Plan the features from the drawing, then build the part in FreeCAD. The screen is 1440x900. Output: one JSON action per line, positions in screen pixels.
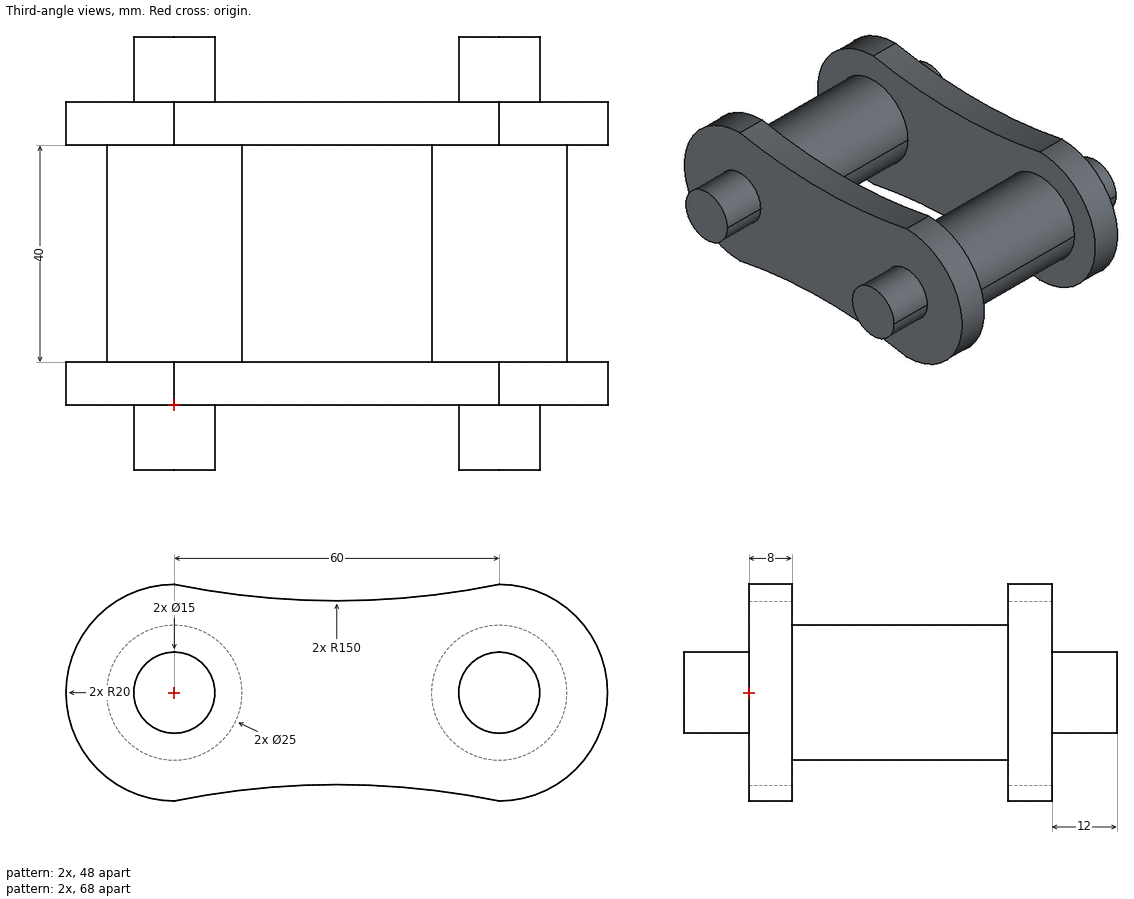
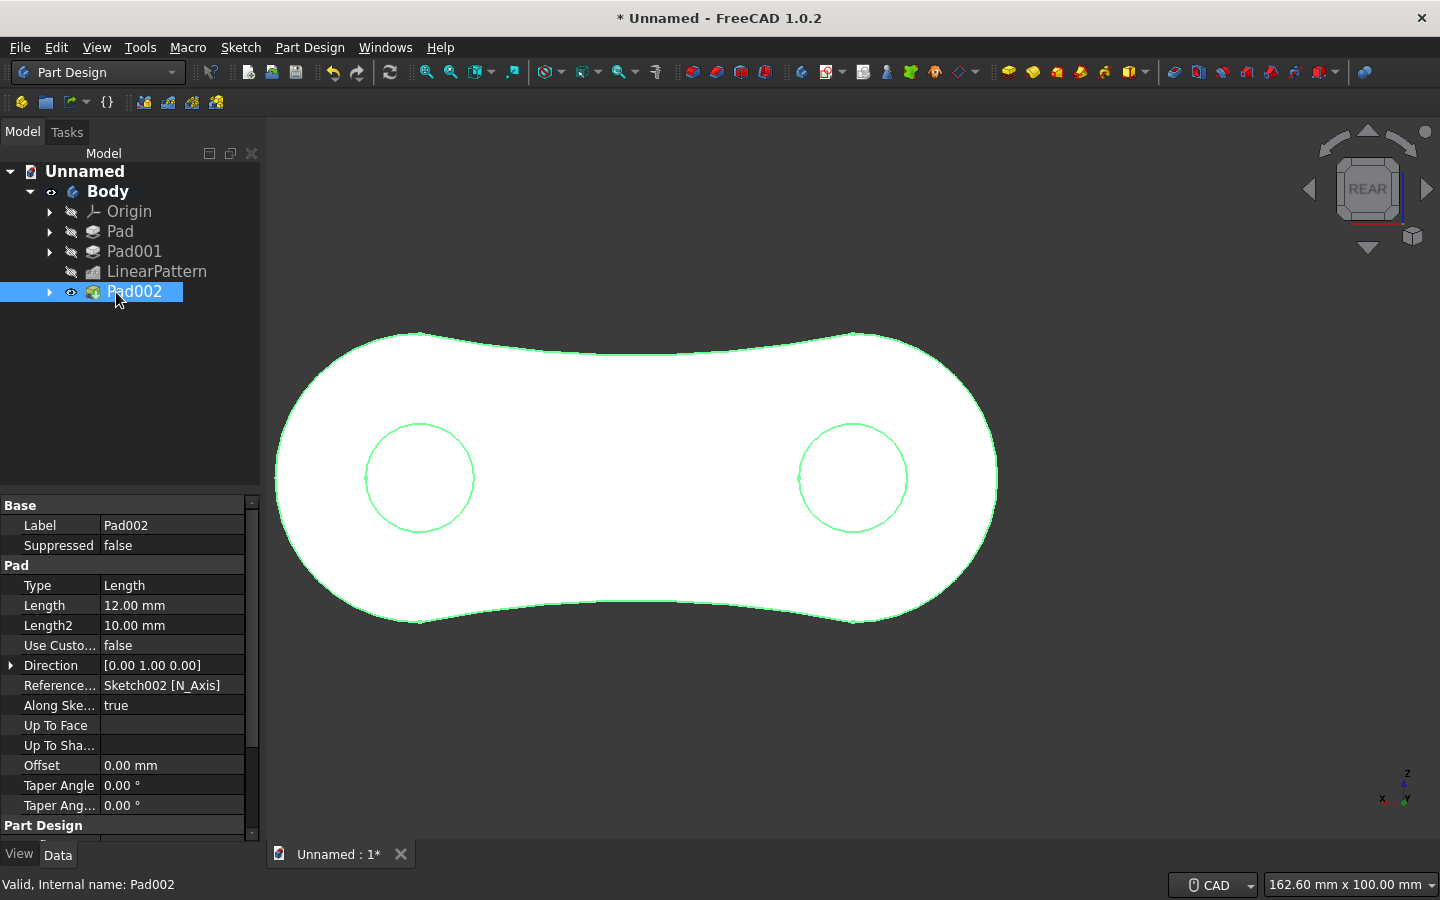
{"action": "left_click", "coordinate": [168, 102]}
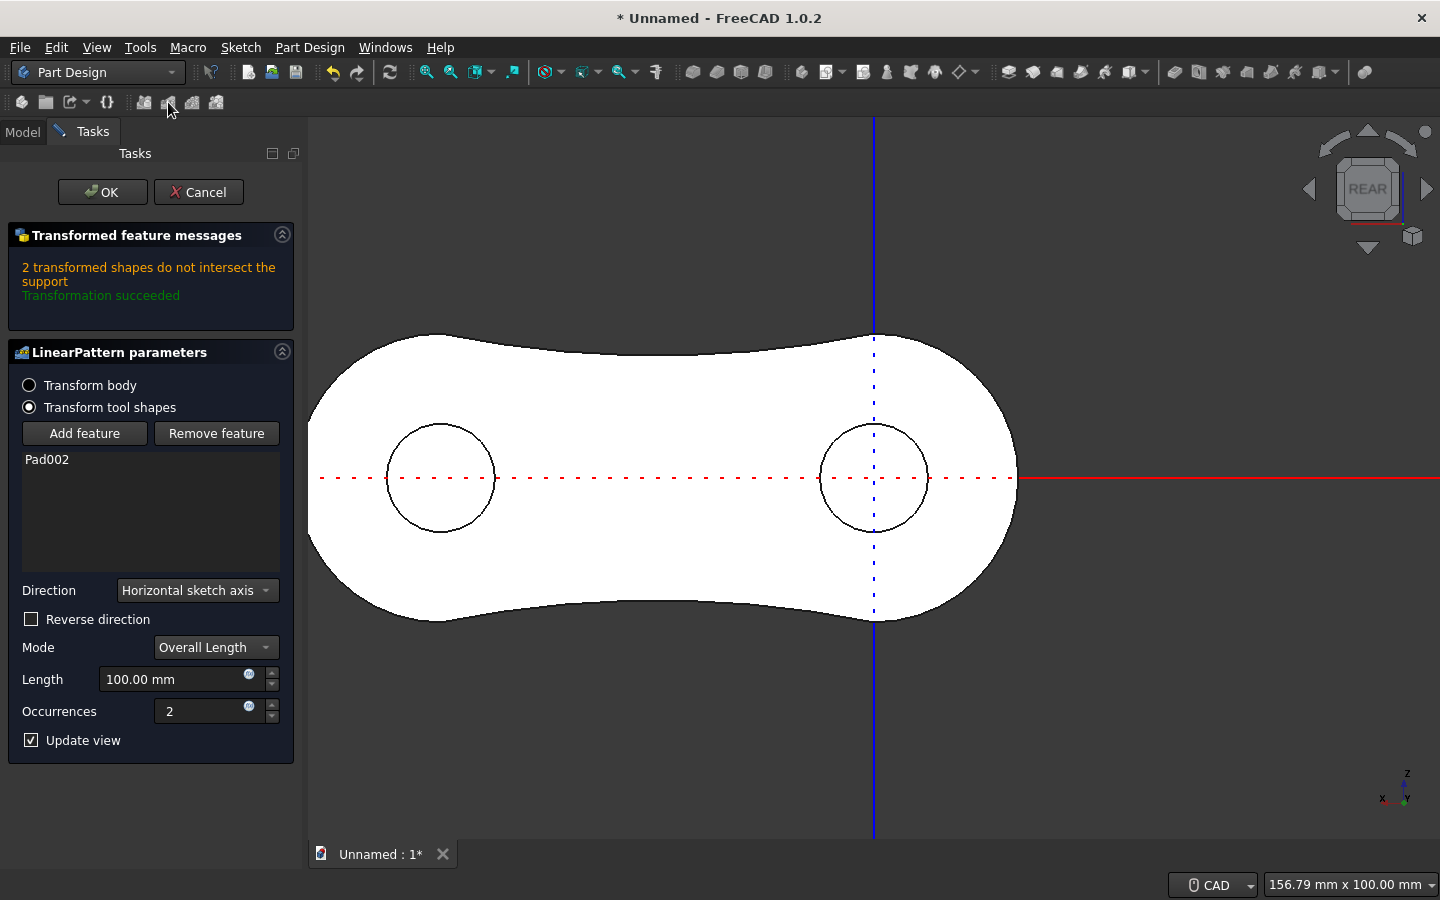
{"action": "left_click", "coordinate": [198, 590]}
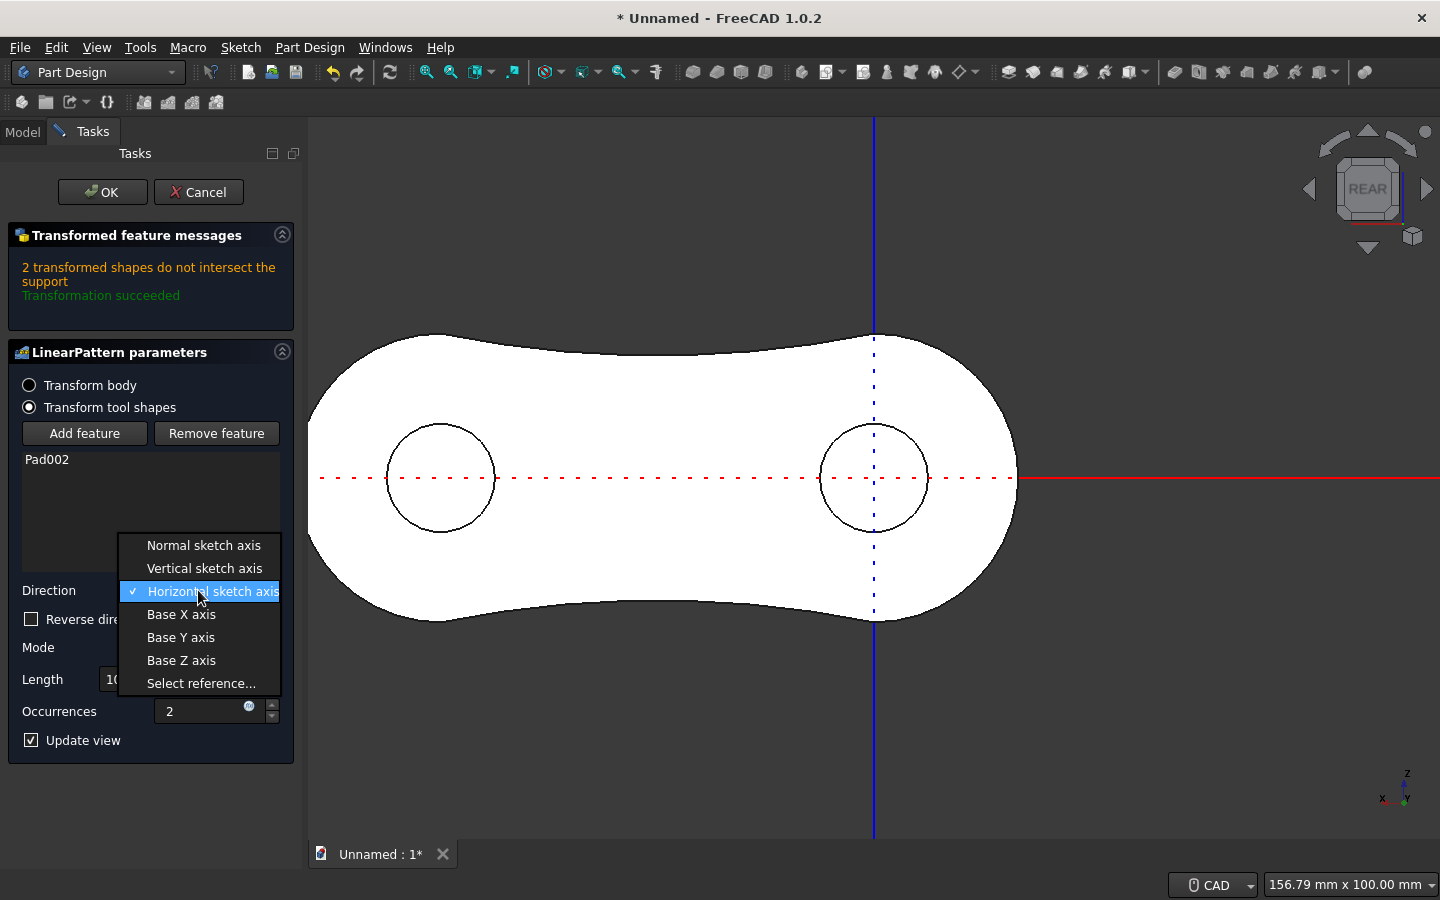
{"action": "left_click", "coordinate": [198, 638]}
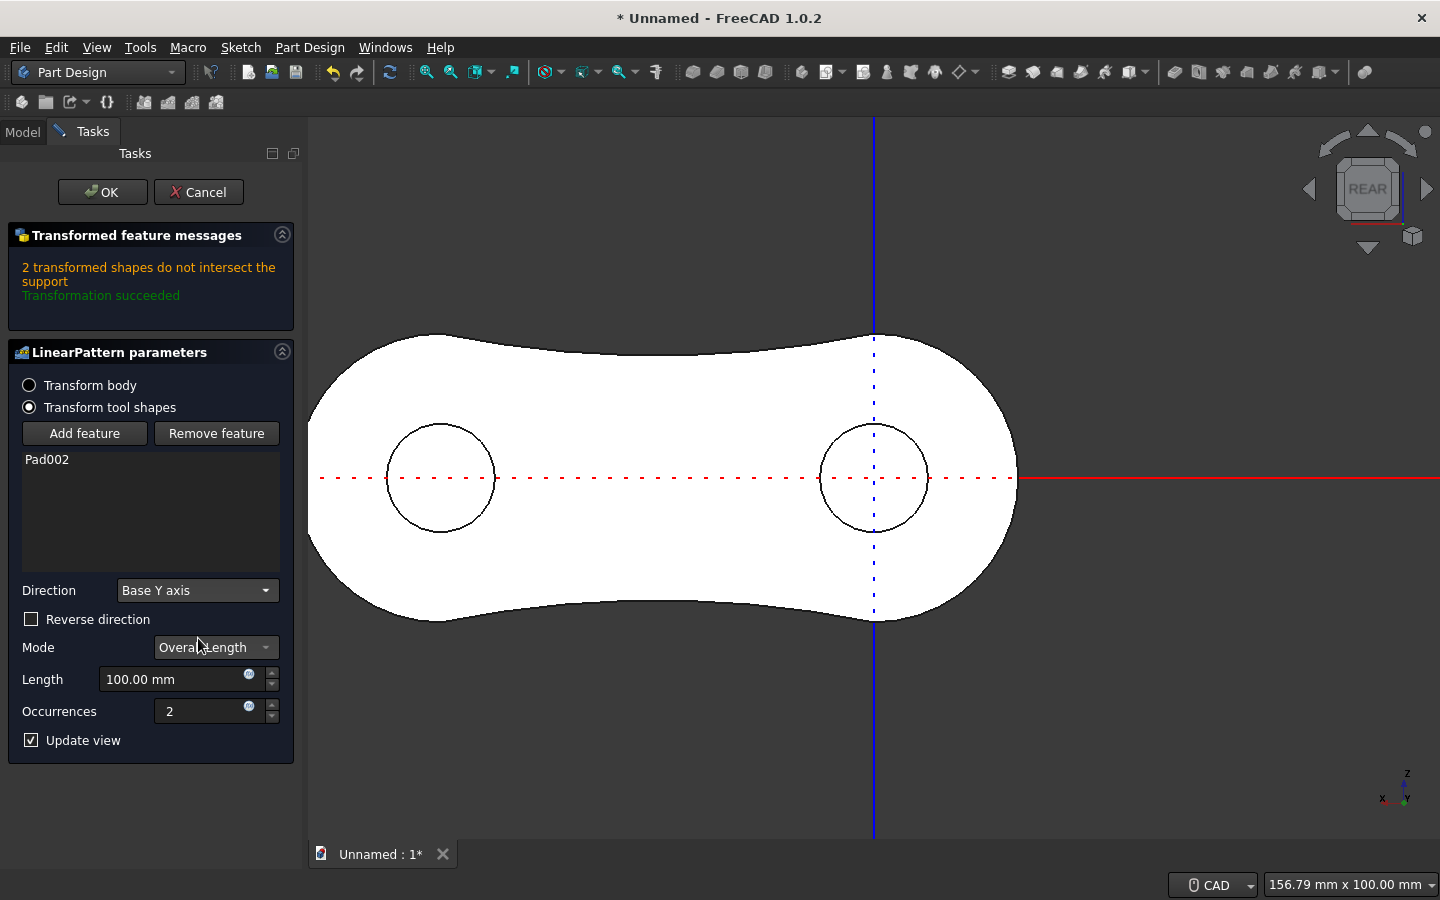
{"action": "left_click", "coordinate": [217, 648]}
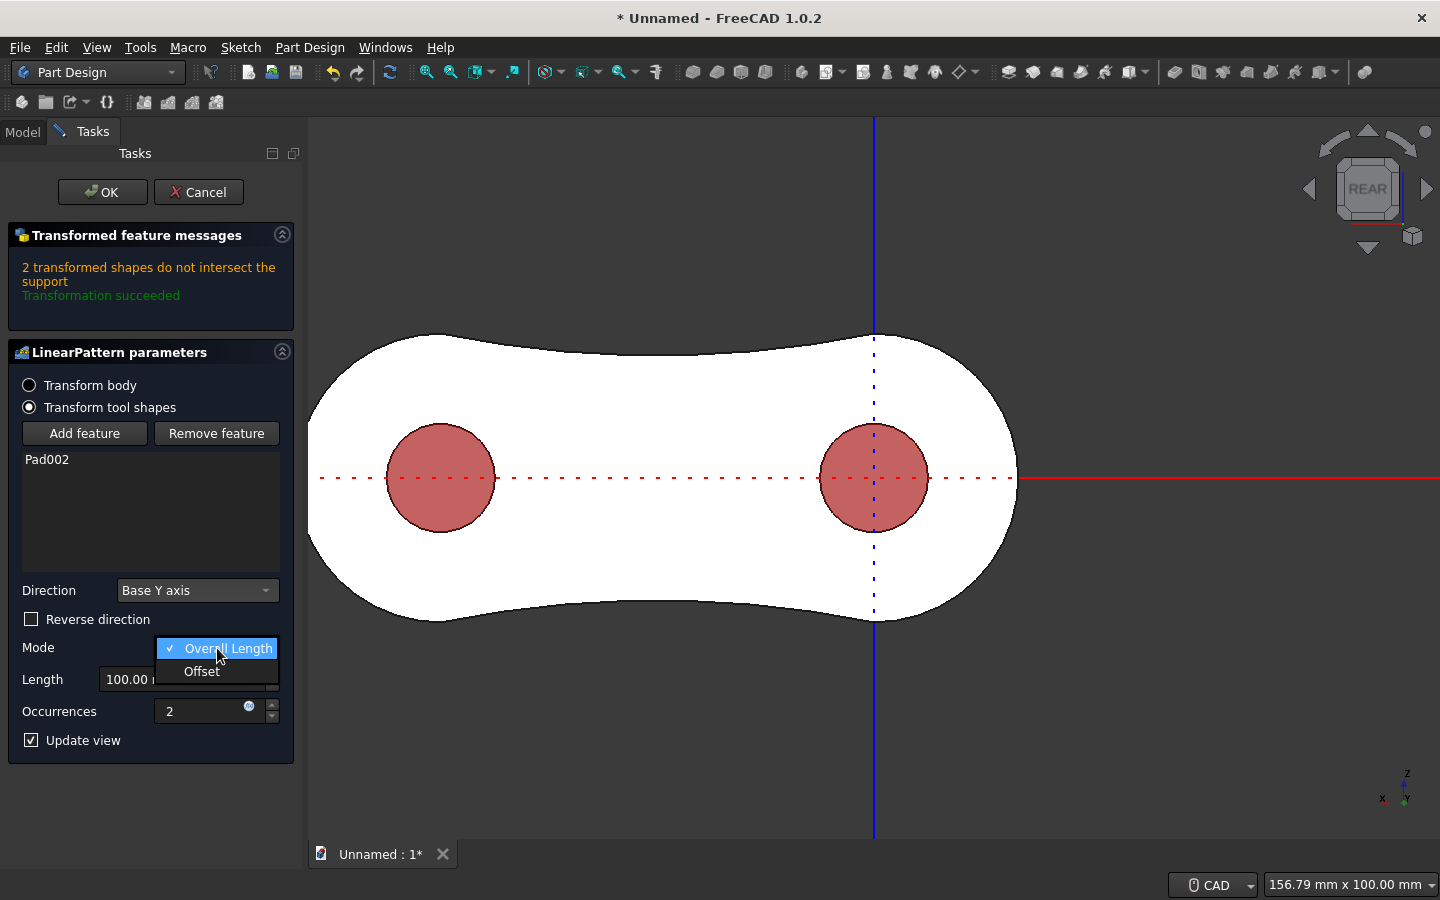
{"action": "left_click", "coordinate": [216, 672]}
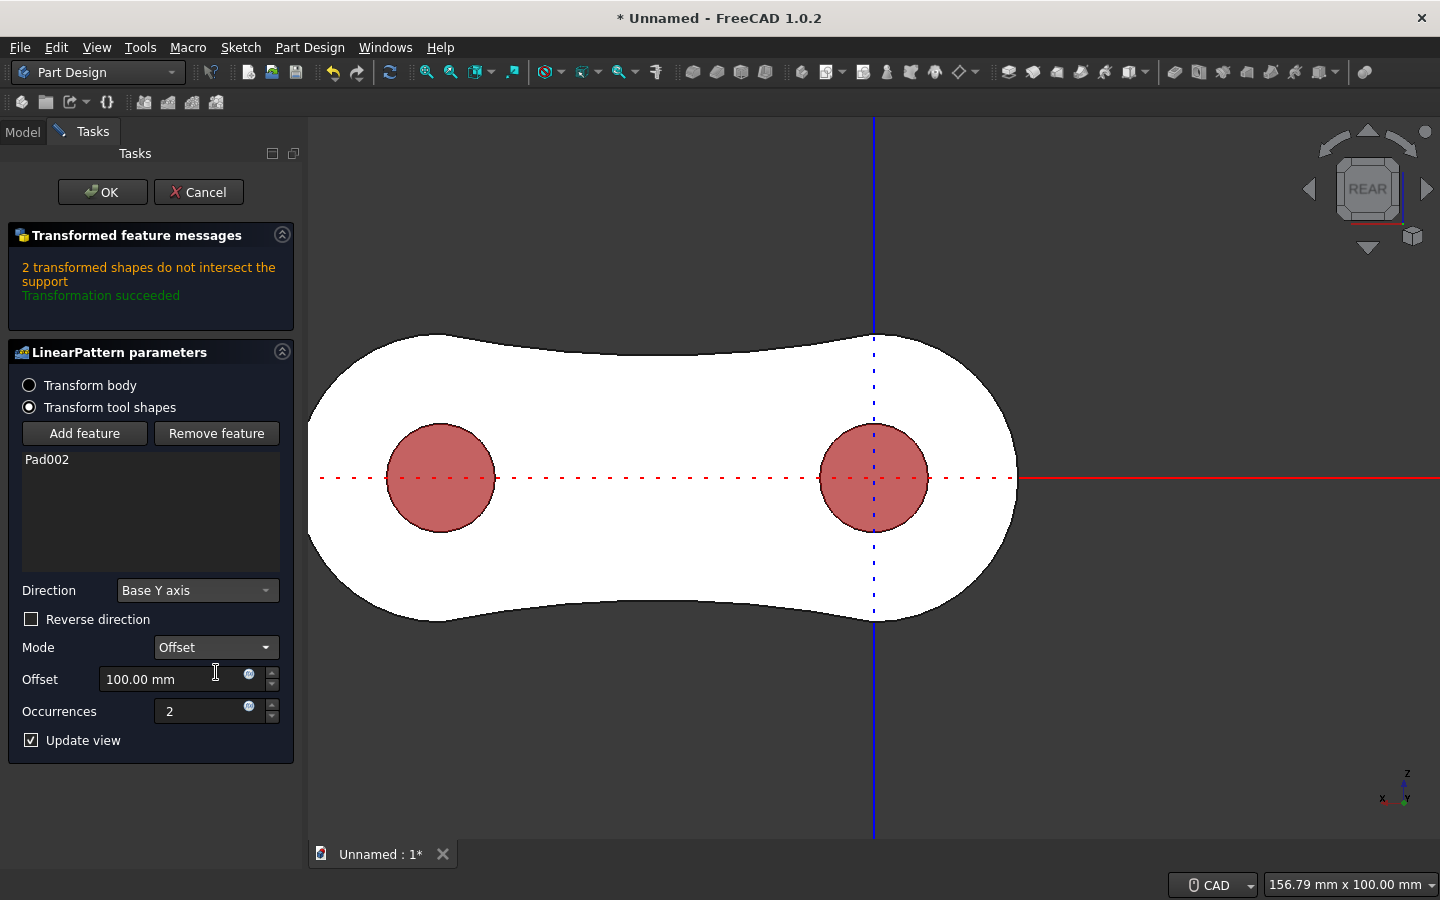
{"action": "triple_click", "coordinate": [182, 679]}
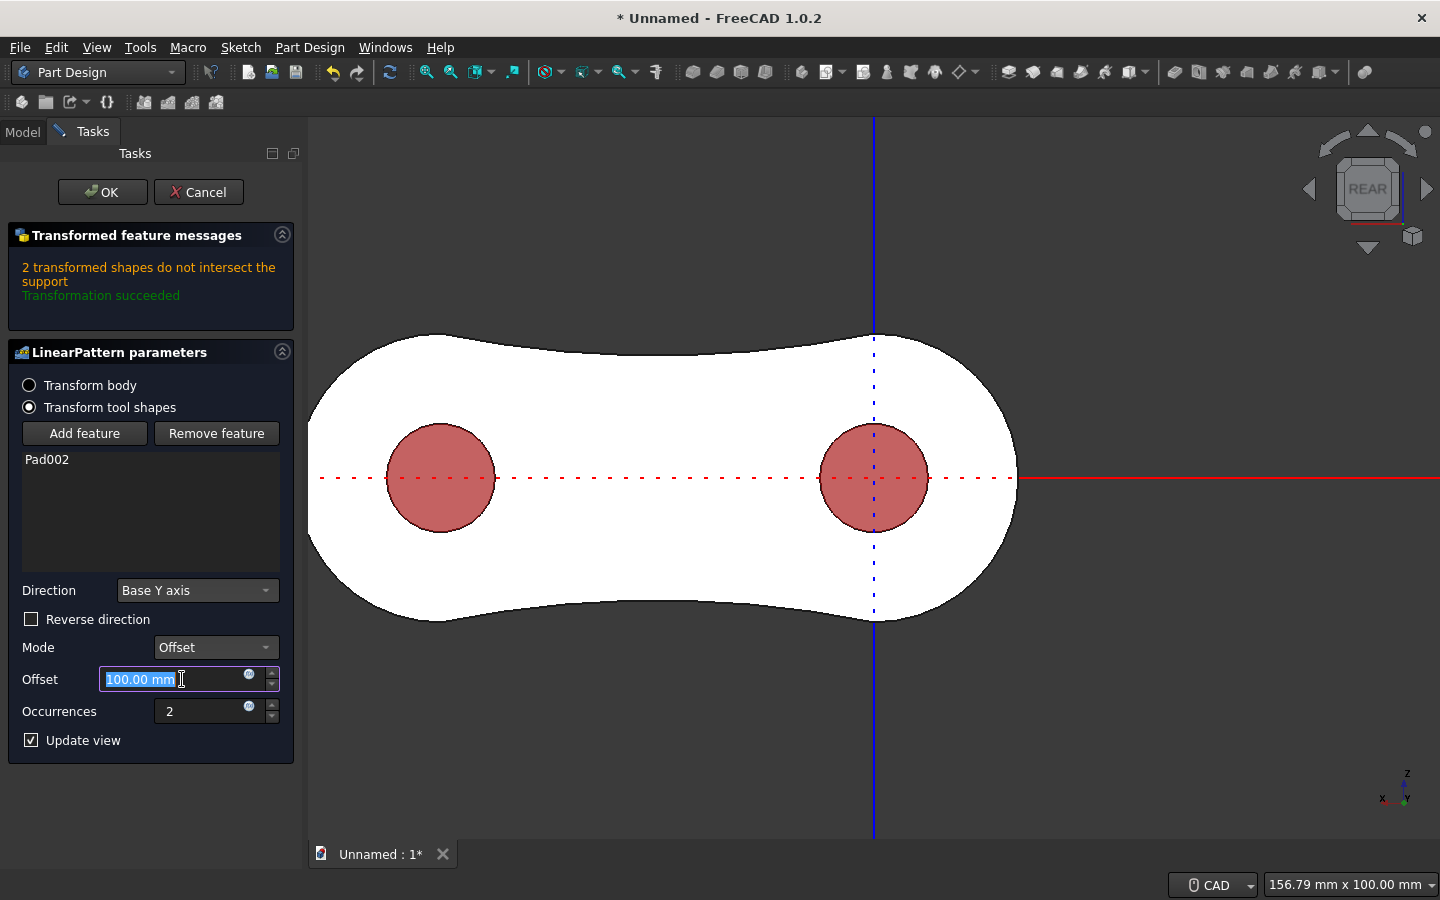
{"action": "type", "text": "68"}
{"action": "key", "text": "Tab"}